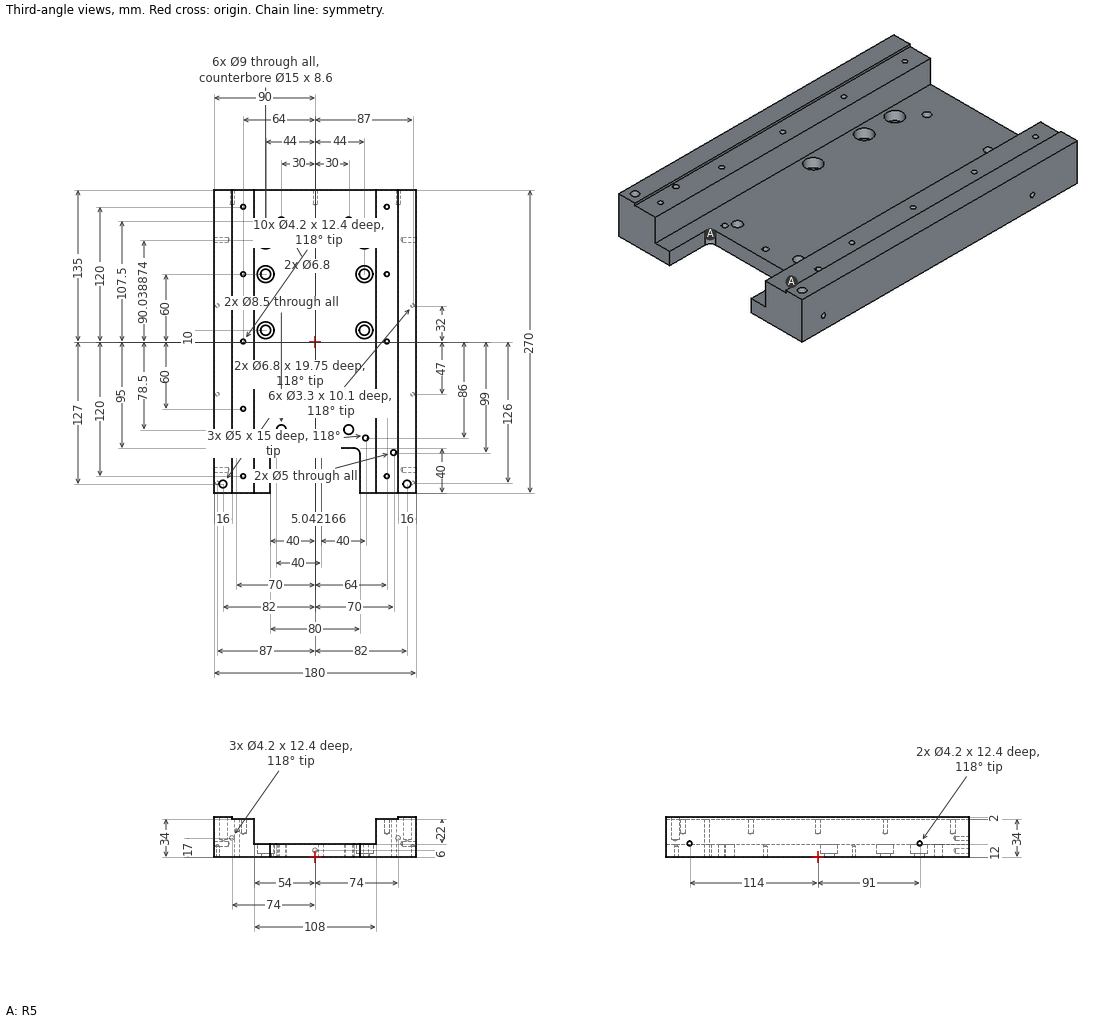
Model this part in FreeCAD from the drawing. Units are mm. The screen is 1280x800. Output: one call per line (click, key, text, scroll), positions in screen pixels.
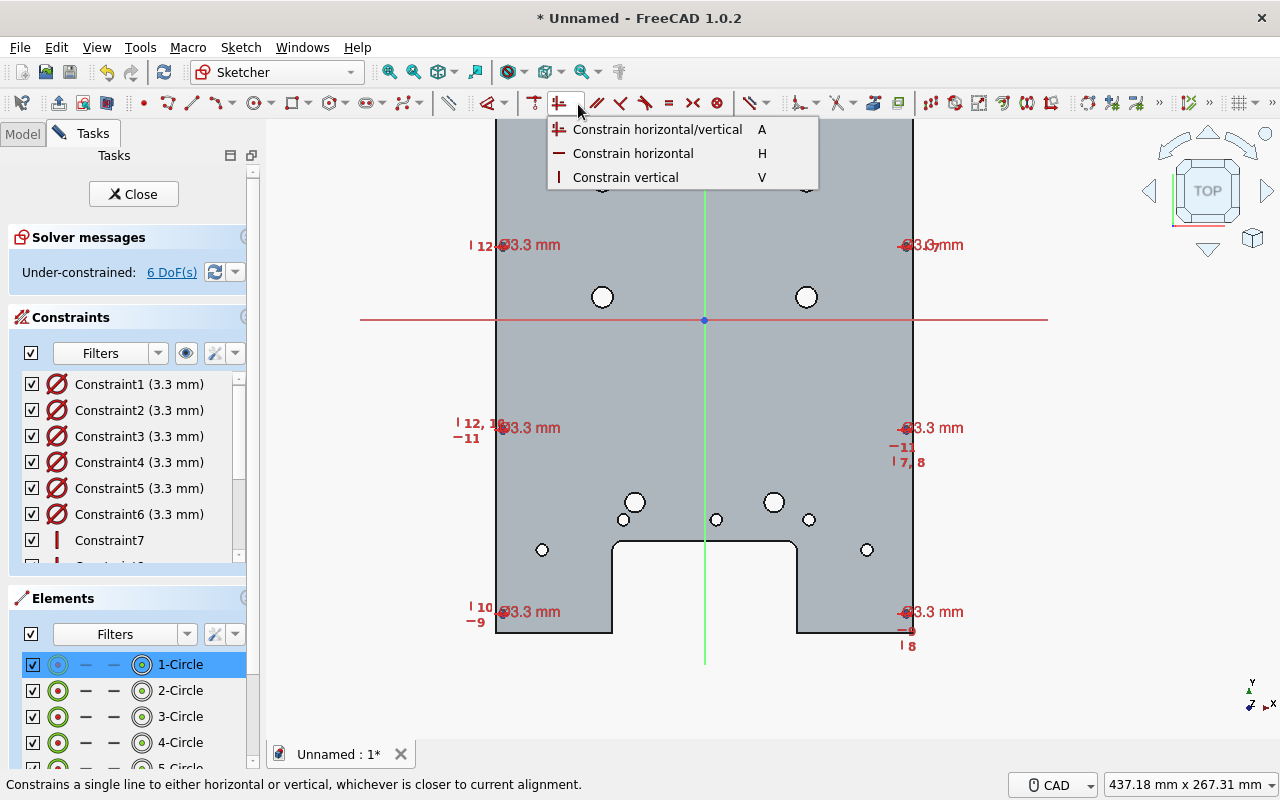
click(683, 153)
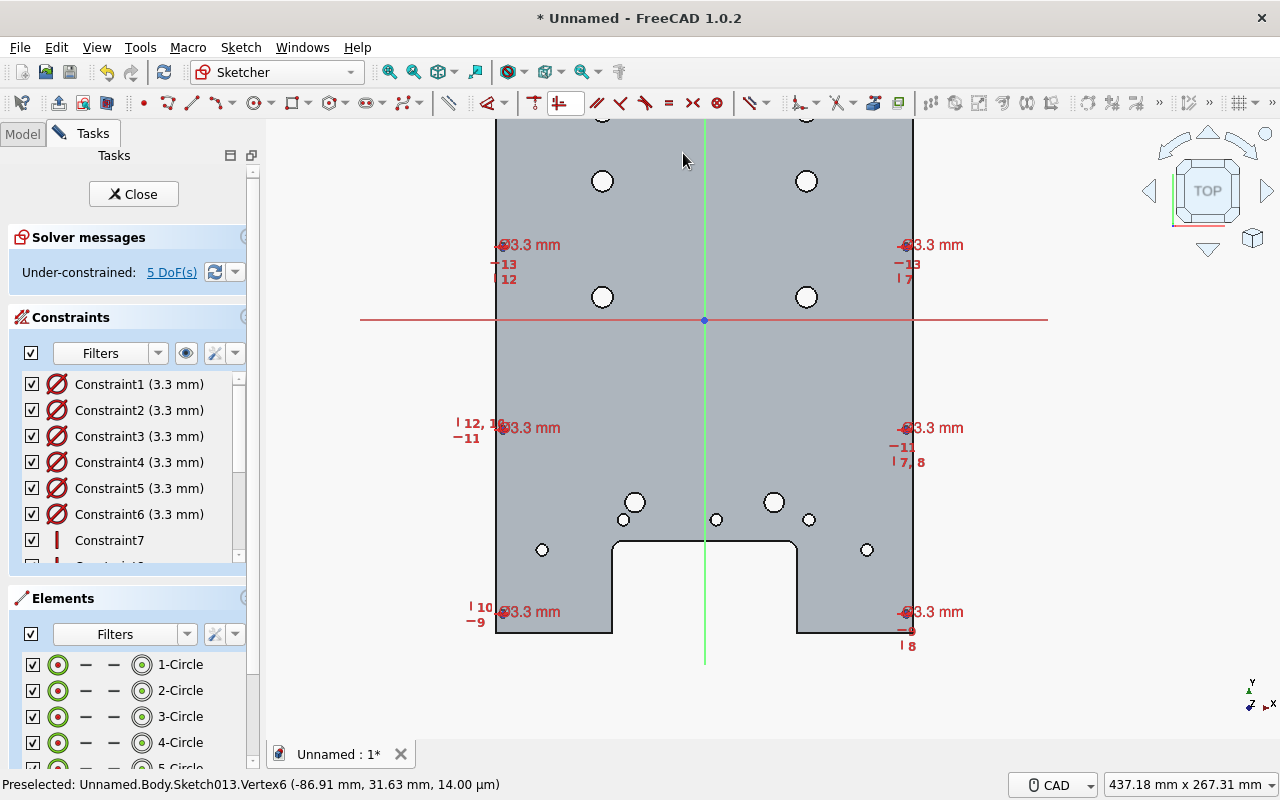
key(d)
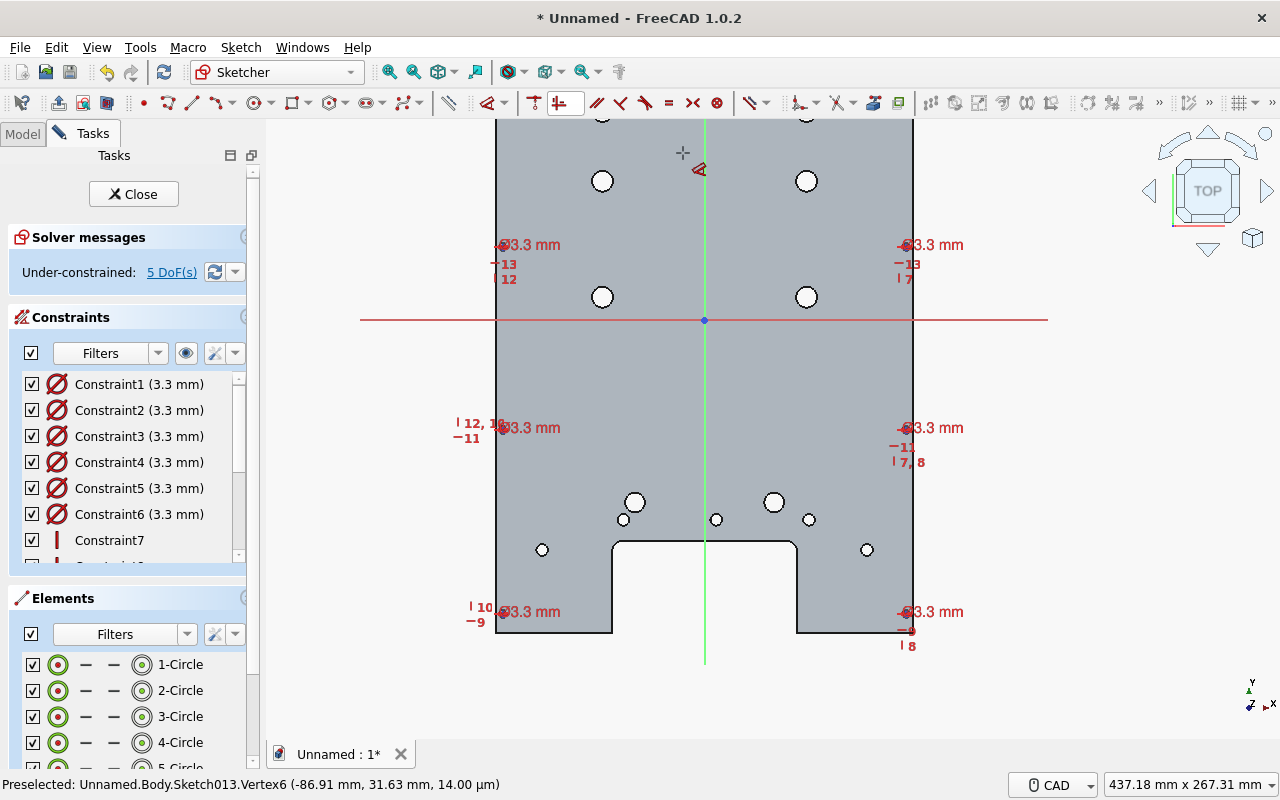
click(906, 247)
click(805, 213)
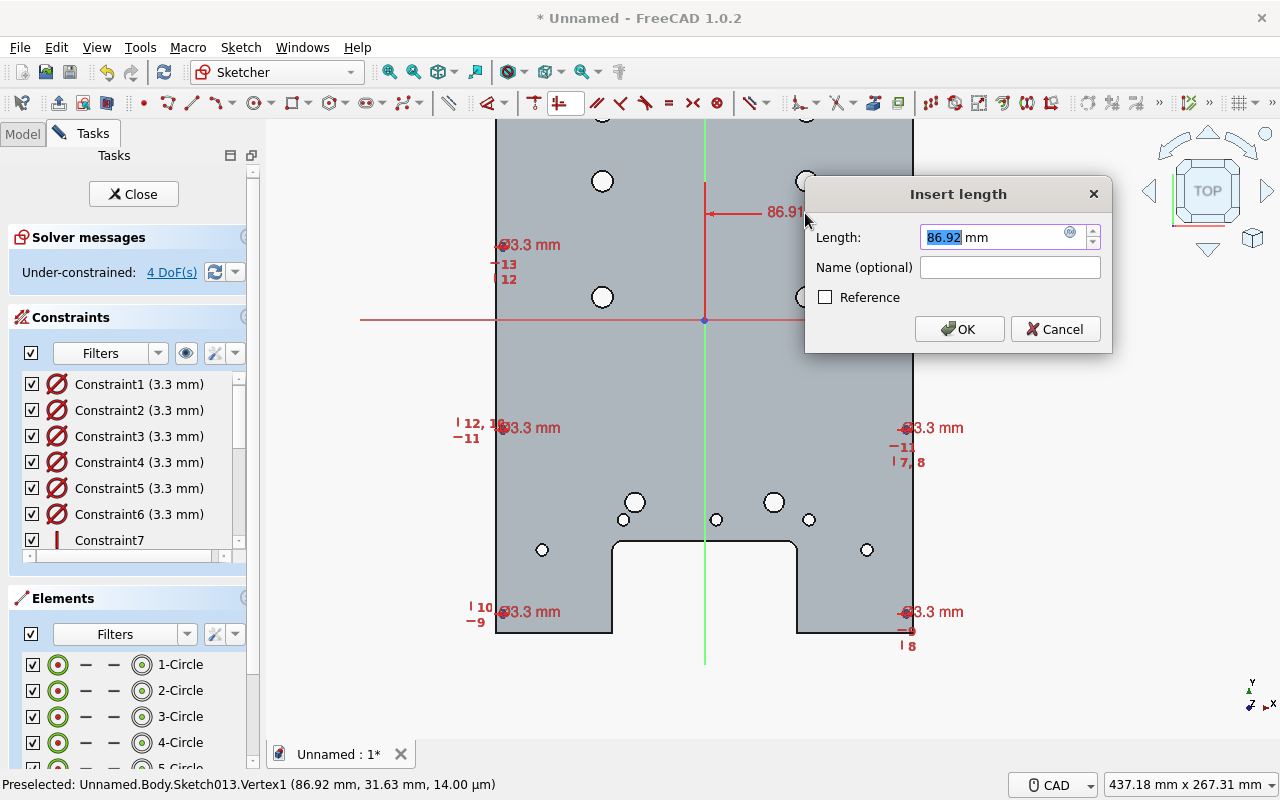
text(87)
key(Return)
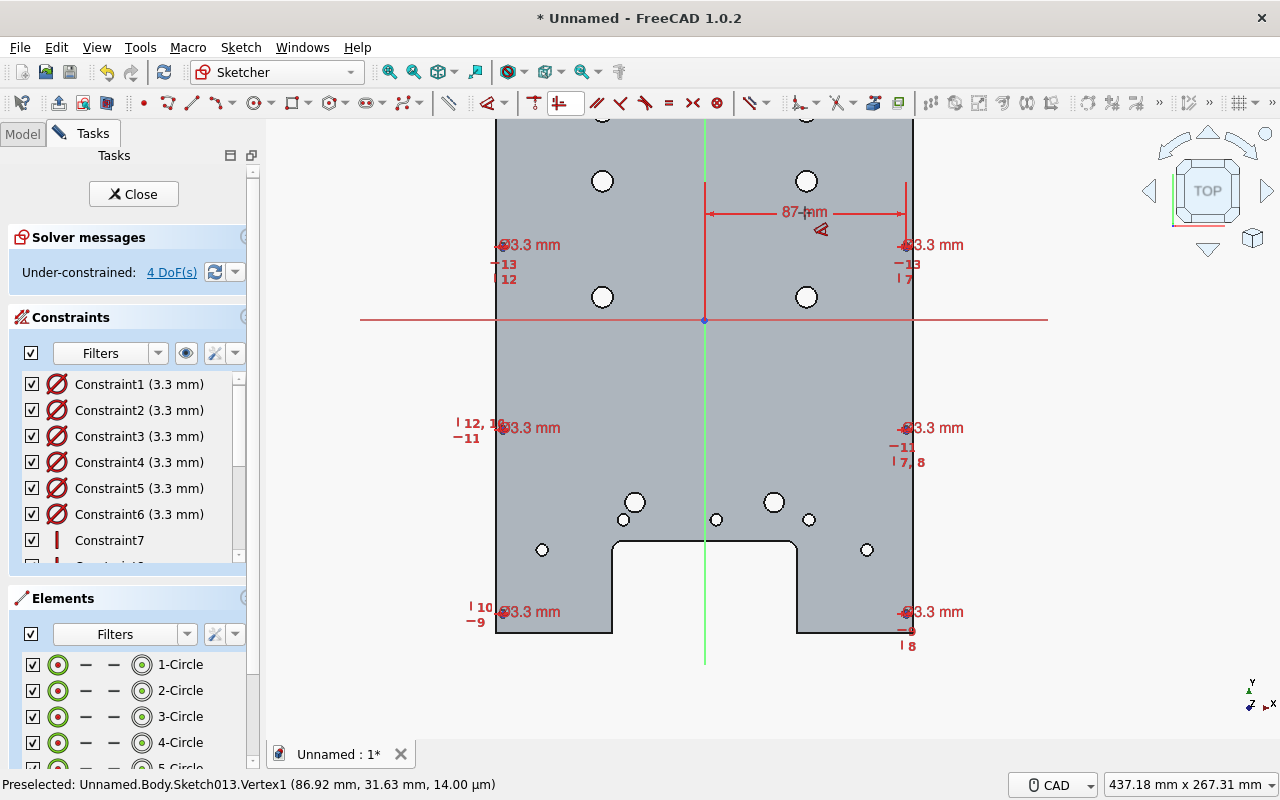
click(906, 247)
click(940, 284)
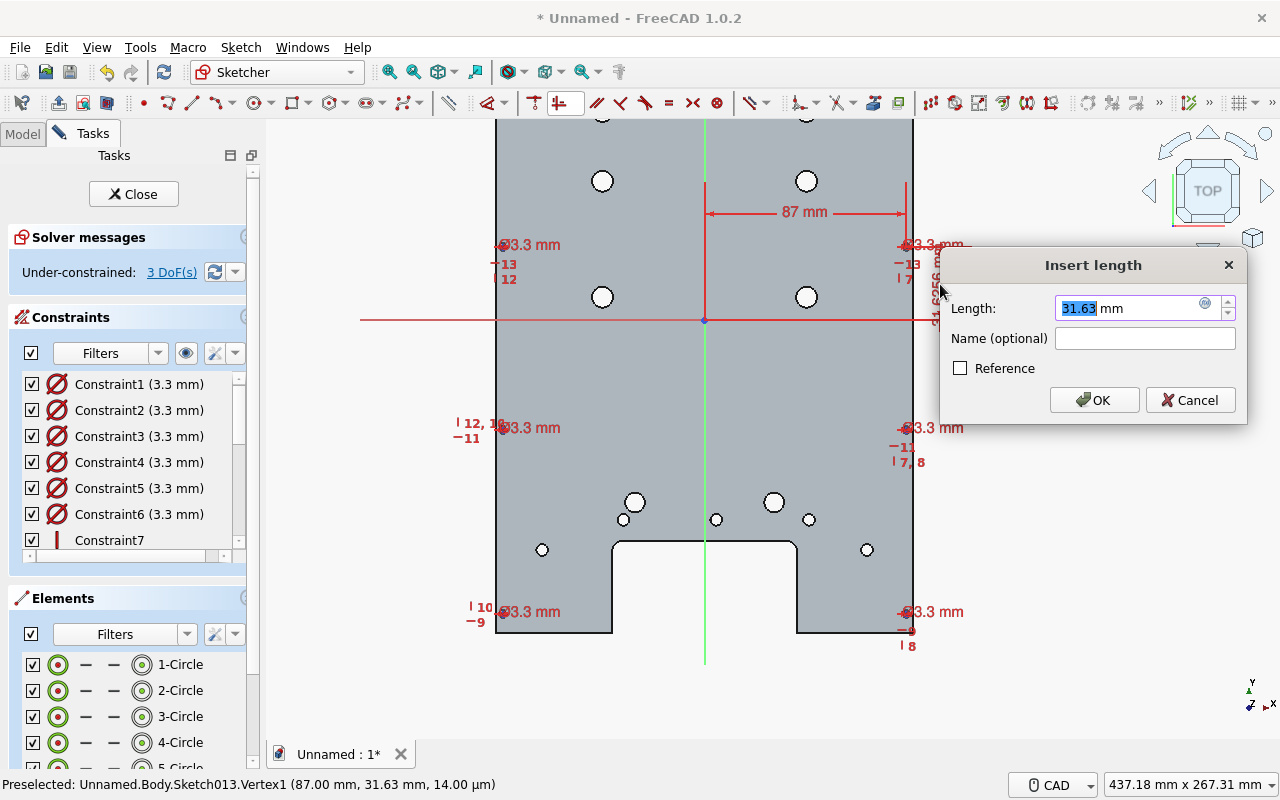
text(32)
key(Return)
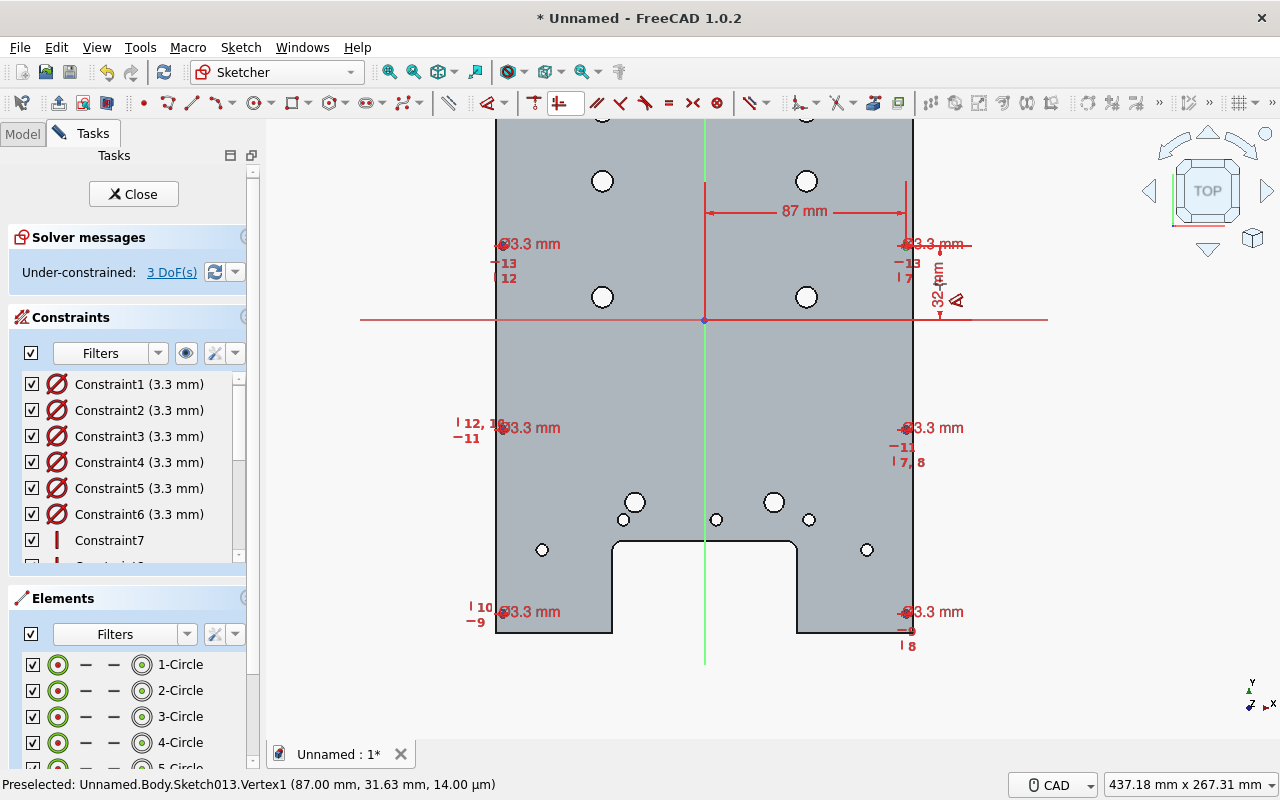
click(906, 430)
click(940, 375)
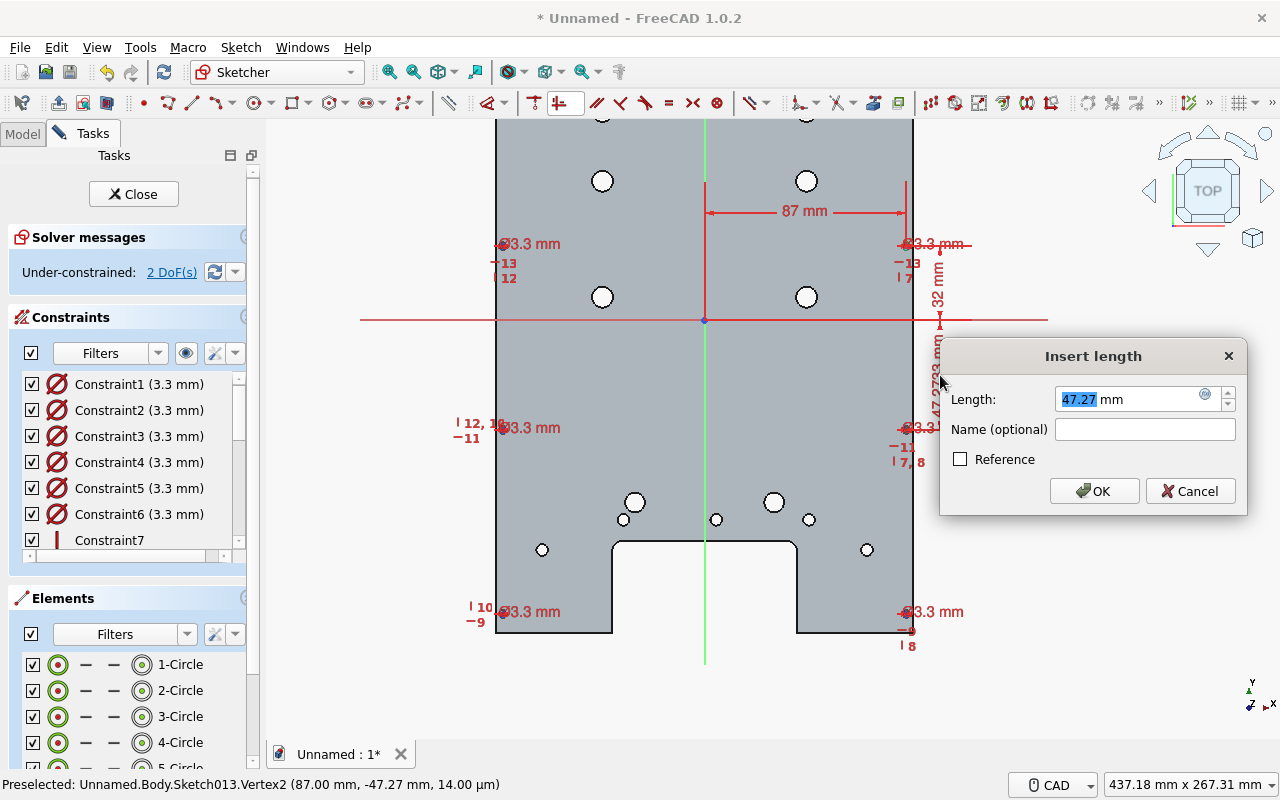
text(47)
key(Return)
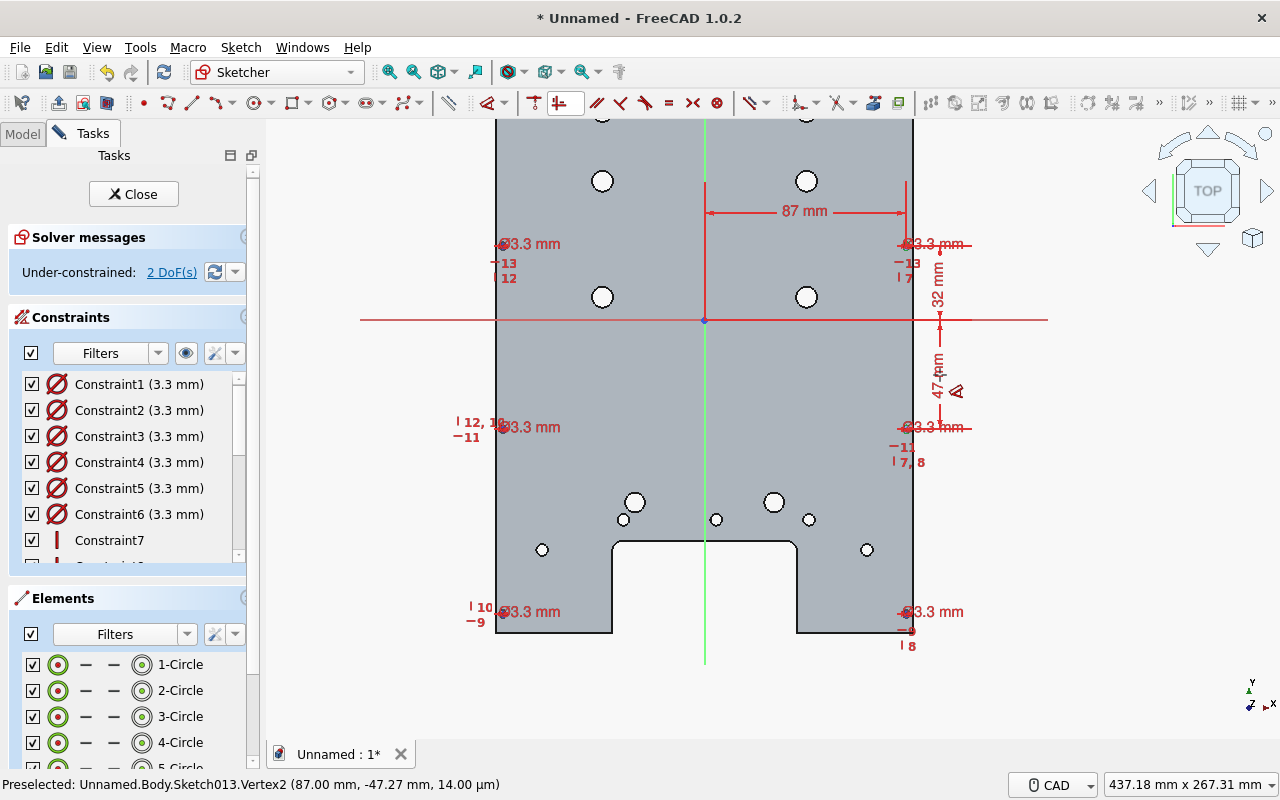
click(503, 614)
click(604, 648)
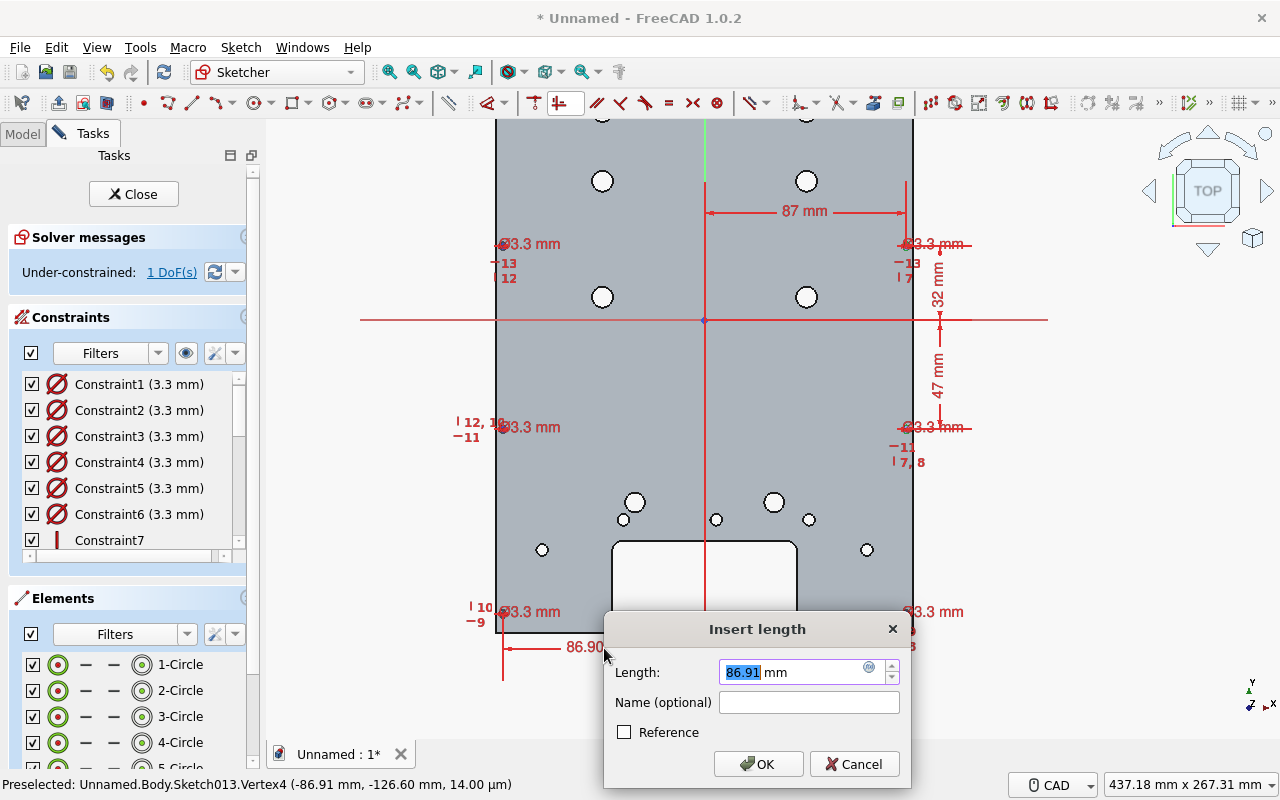
text(87)
key(Return)